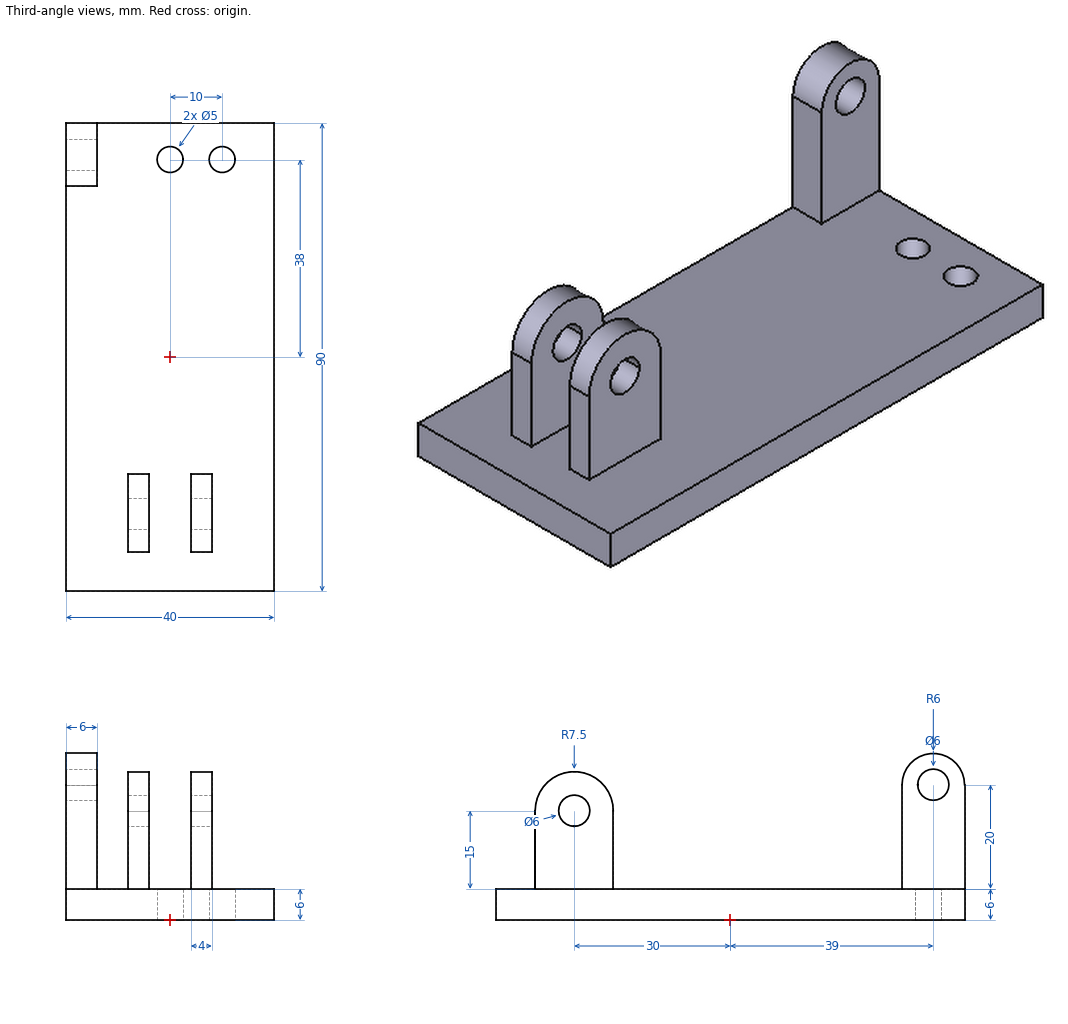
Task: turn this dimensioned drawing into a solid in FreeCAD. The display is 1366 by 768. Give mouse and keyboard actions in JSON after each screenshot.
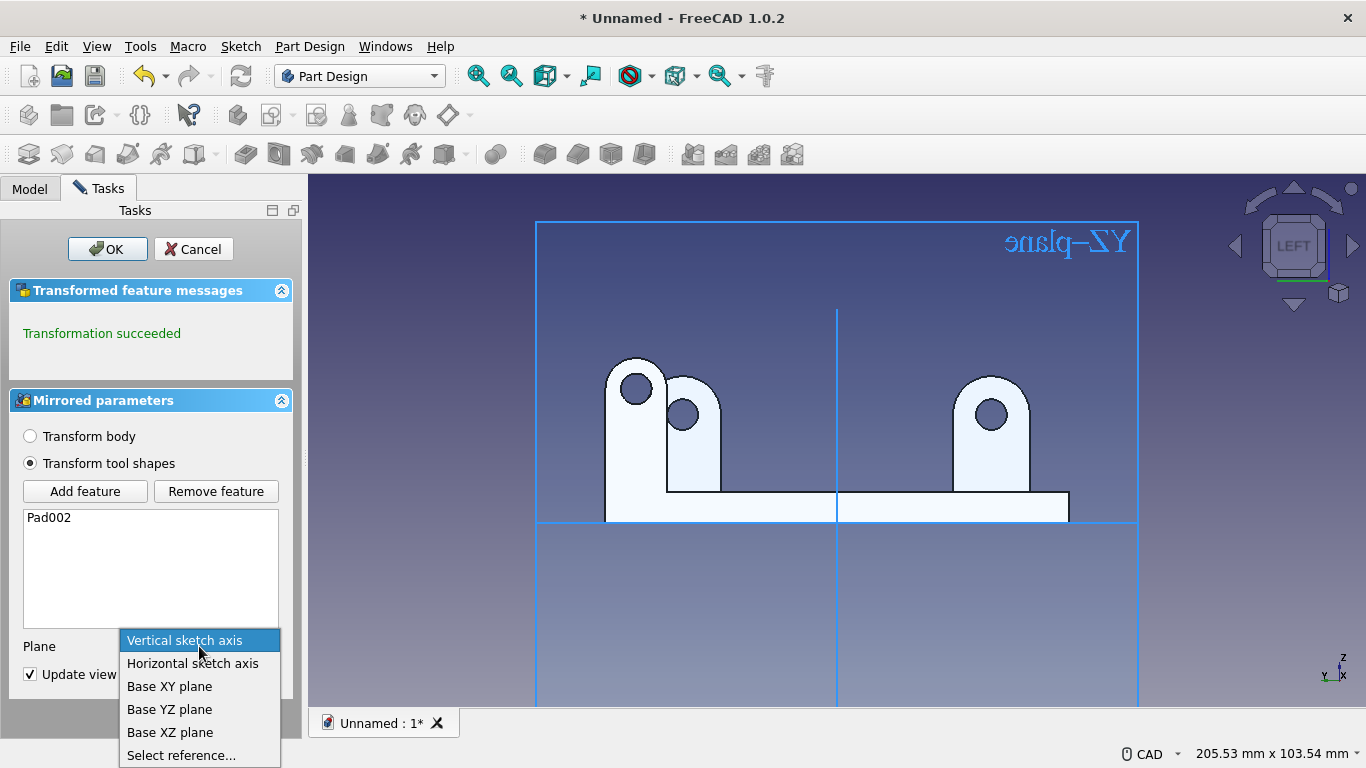
{"action": "left_click", "coordinate": [198, 710]}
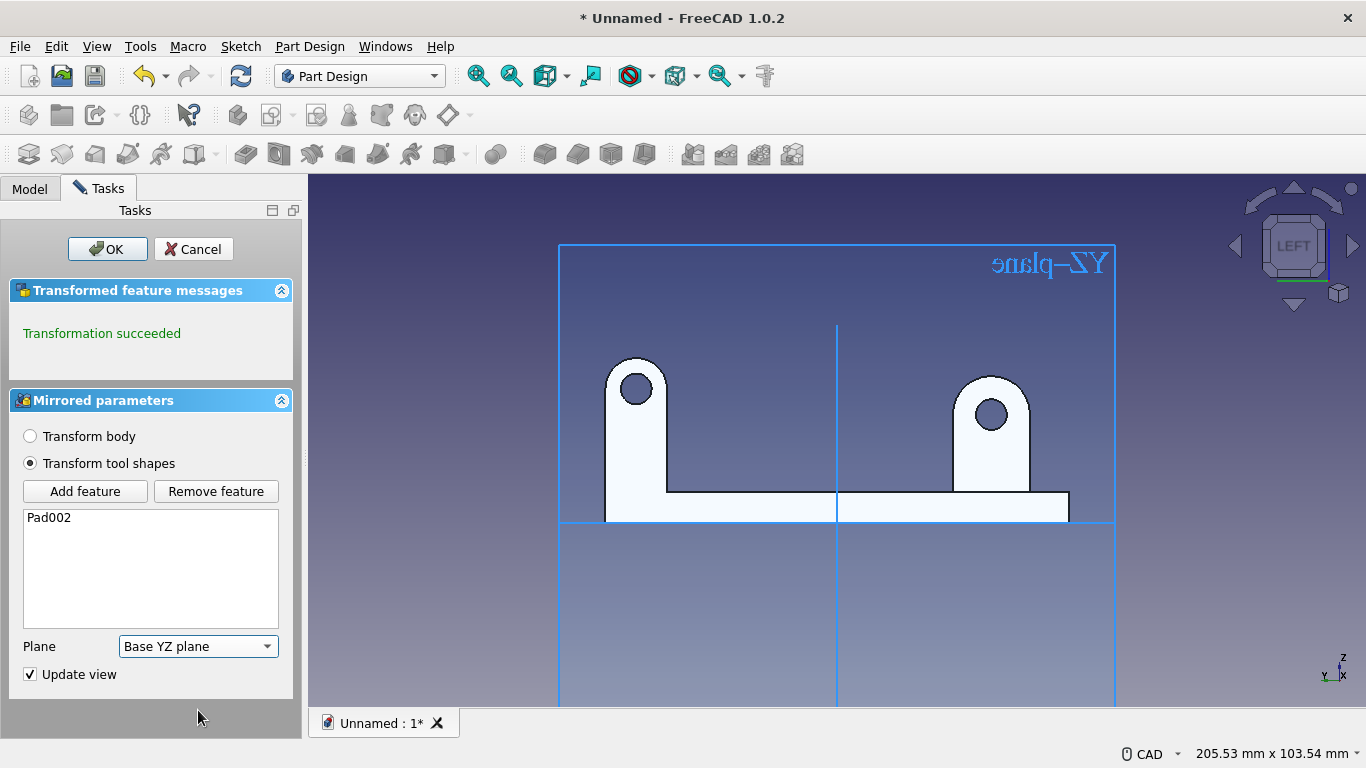
{"action": "left_click", "coordinate": [108, 249]}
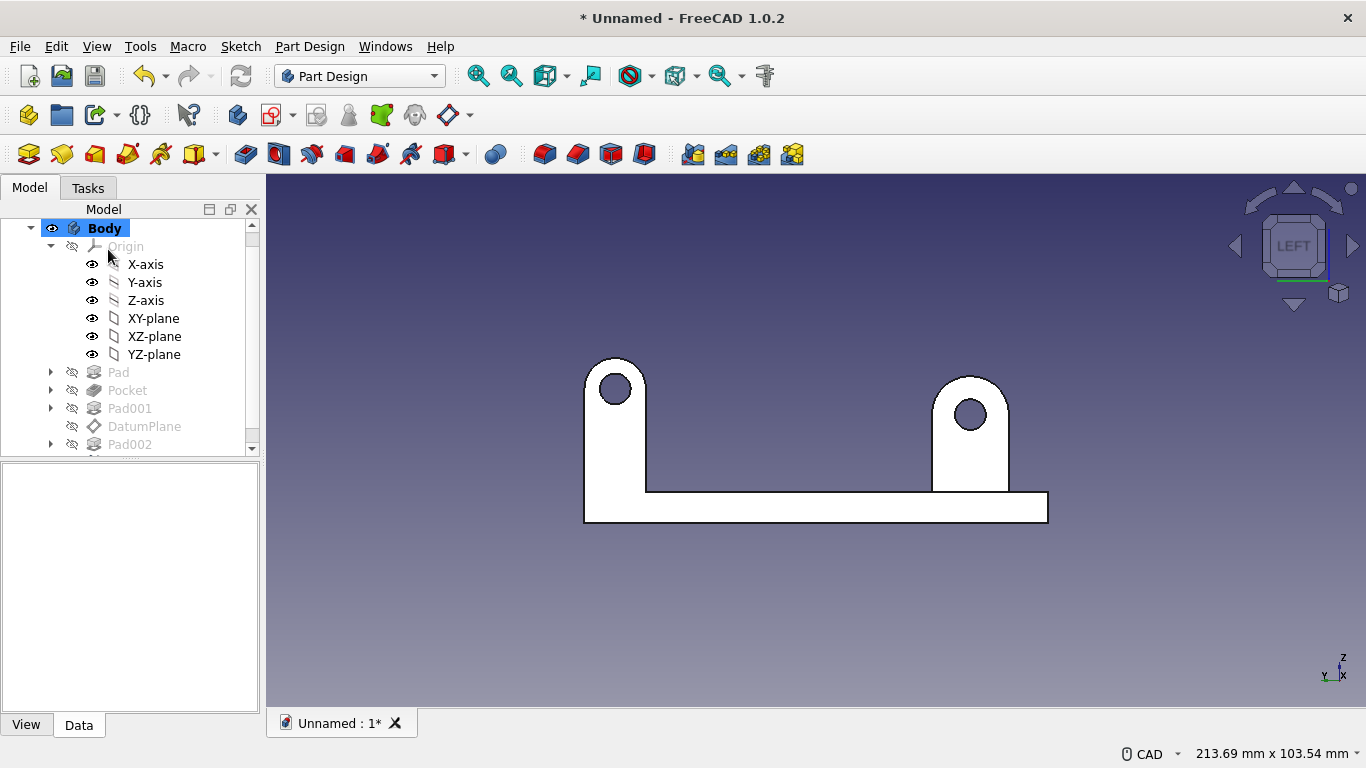
{"action": "key", "text": "0"}